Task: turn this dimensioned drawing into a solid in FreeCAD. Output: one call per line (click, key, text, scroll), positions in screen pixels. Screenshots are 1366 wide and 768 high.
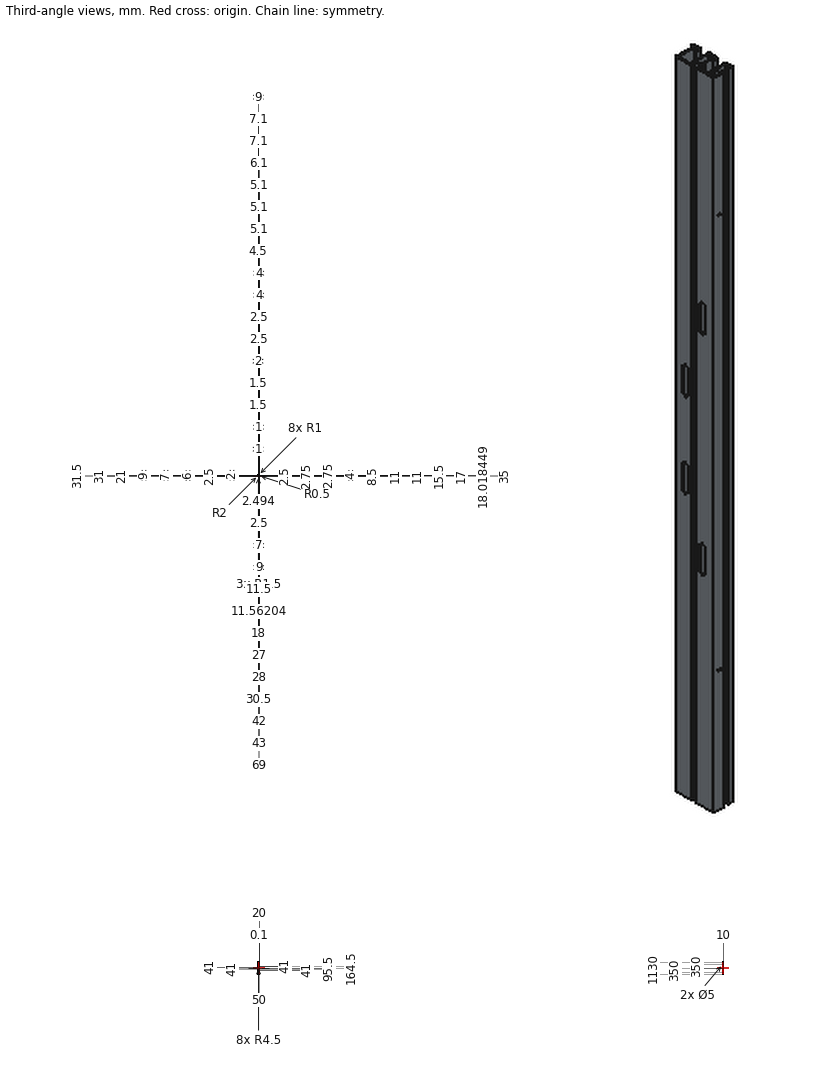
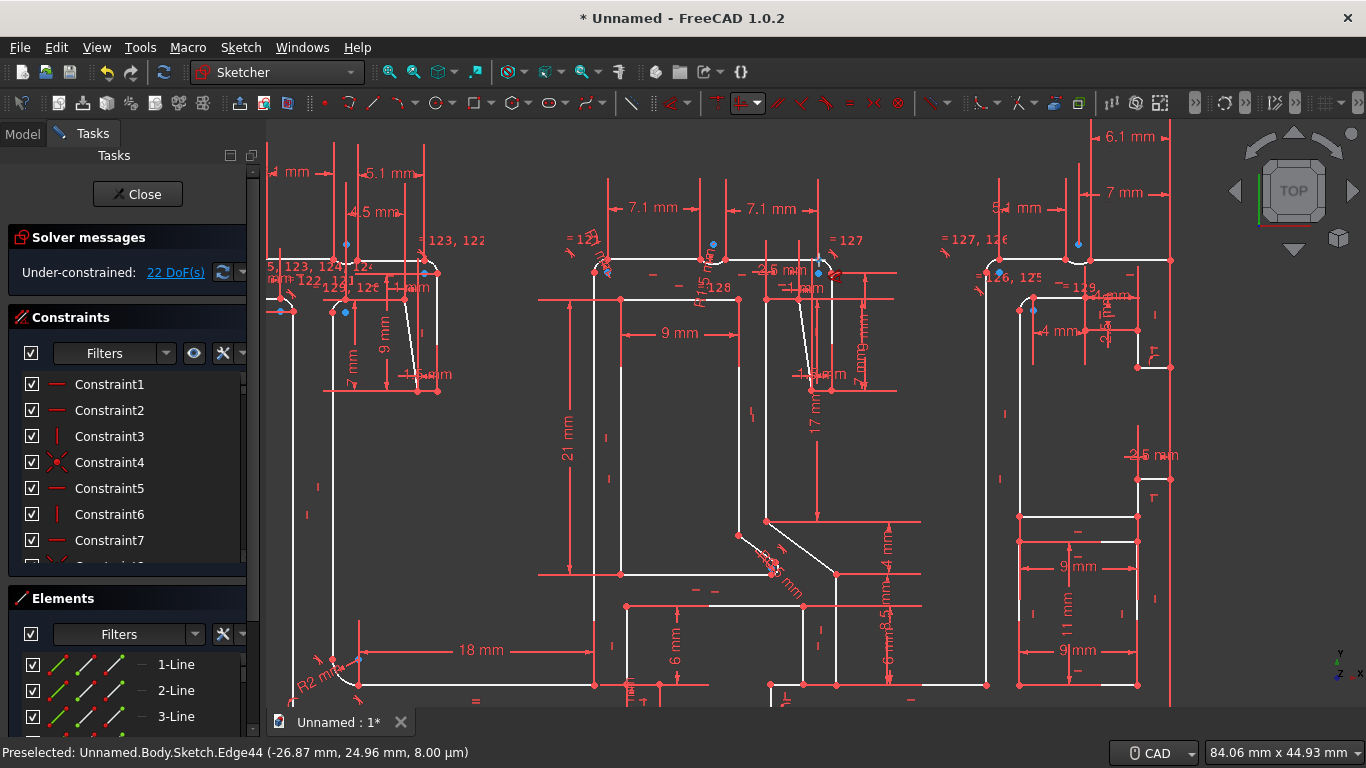
click(818, 260)
click(914, 226)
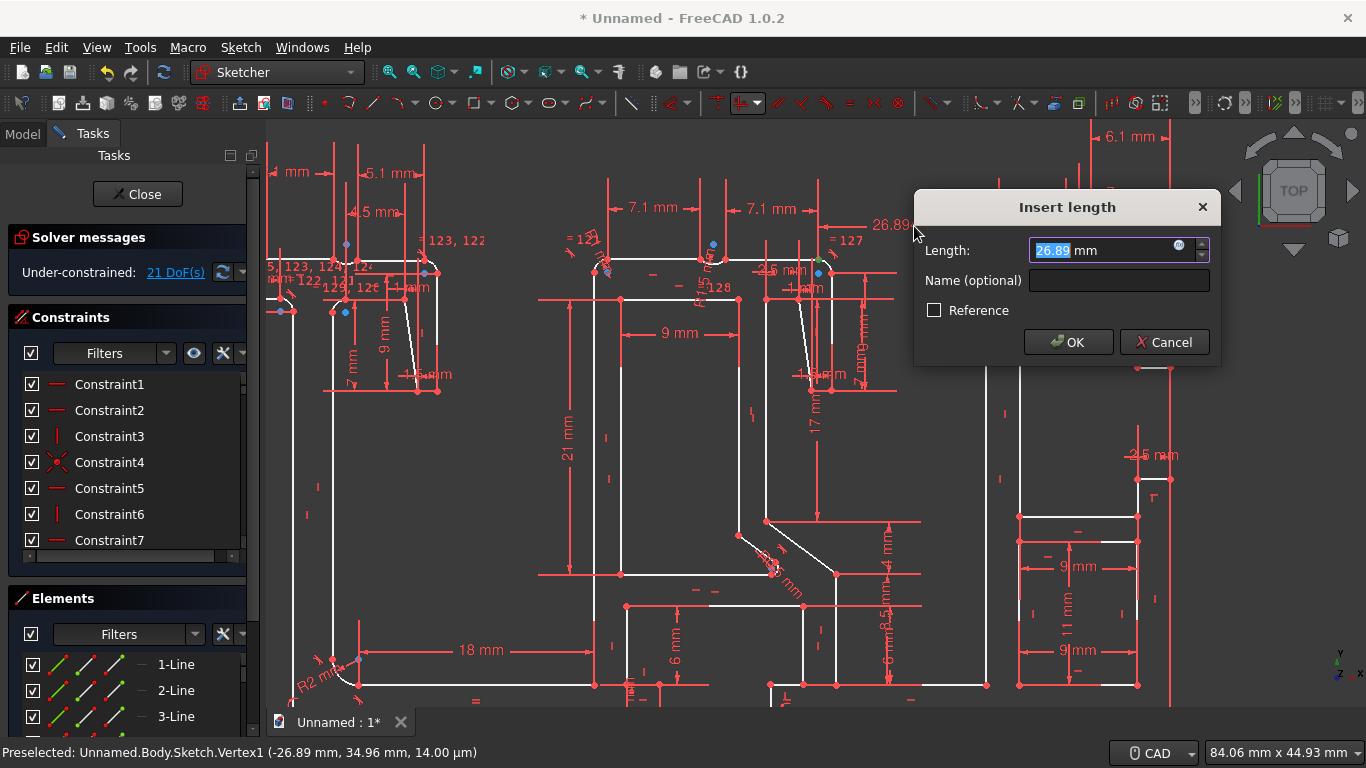
text(27)
key(Return)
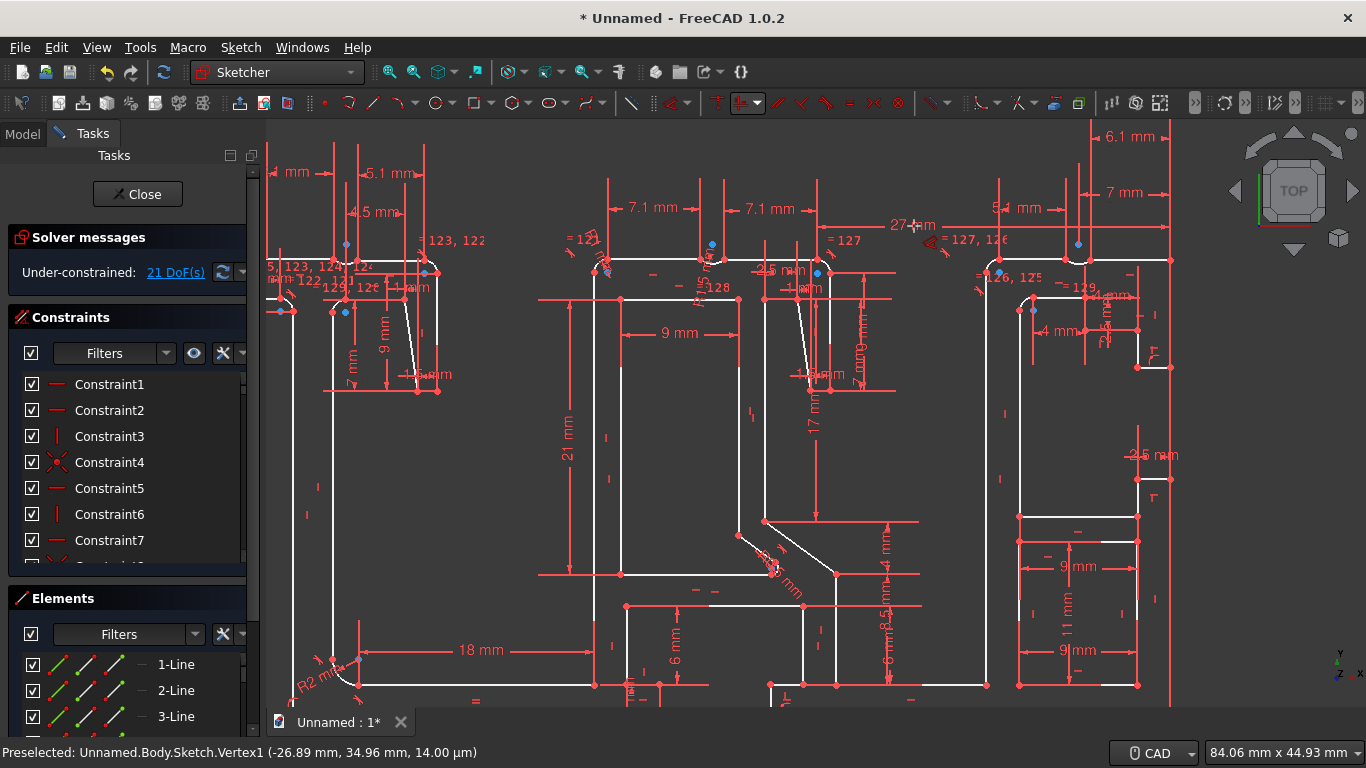
click(817, 260)
click(783, 469)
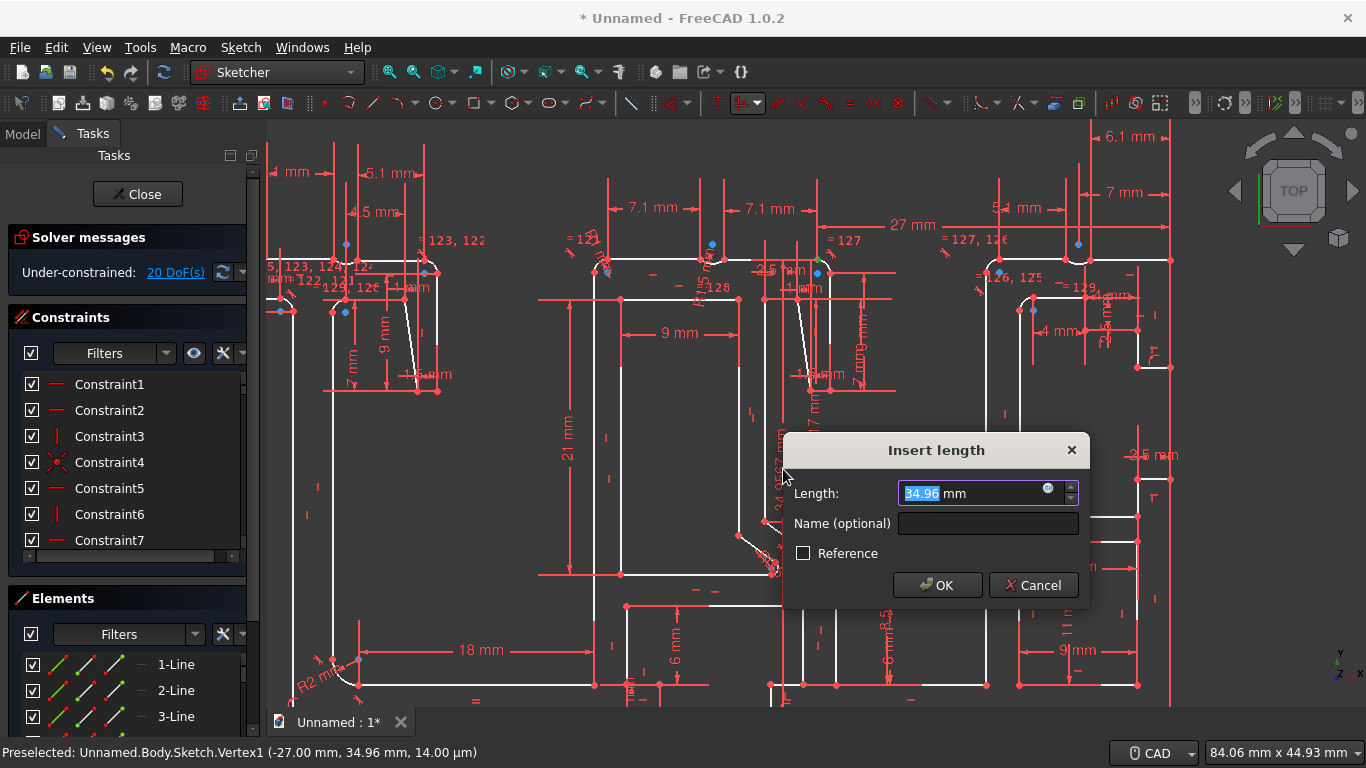
text(35)
key(Return)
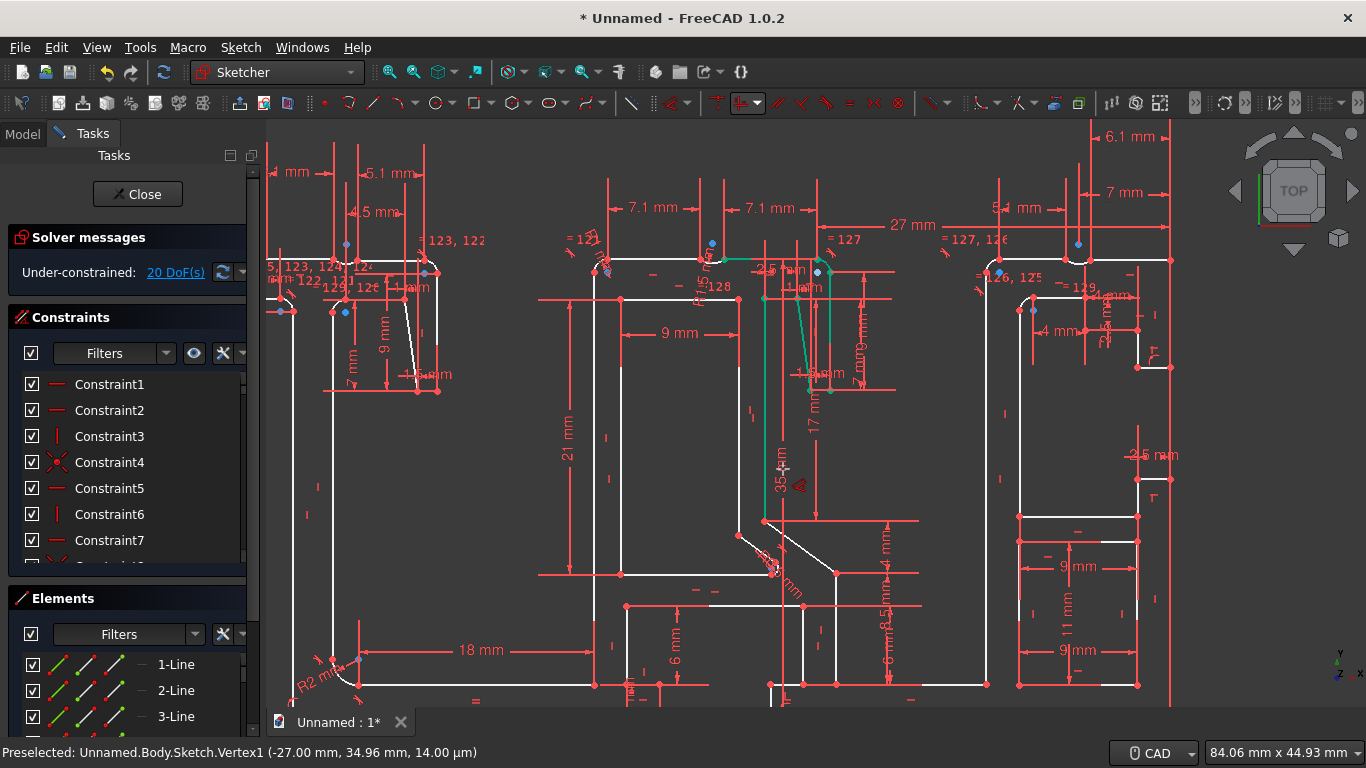
click(700, 259)
click(666, 469)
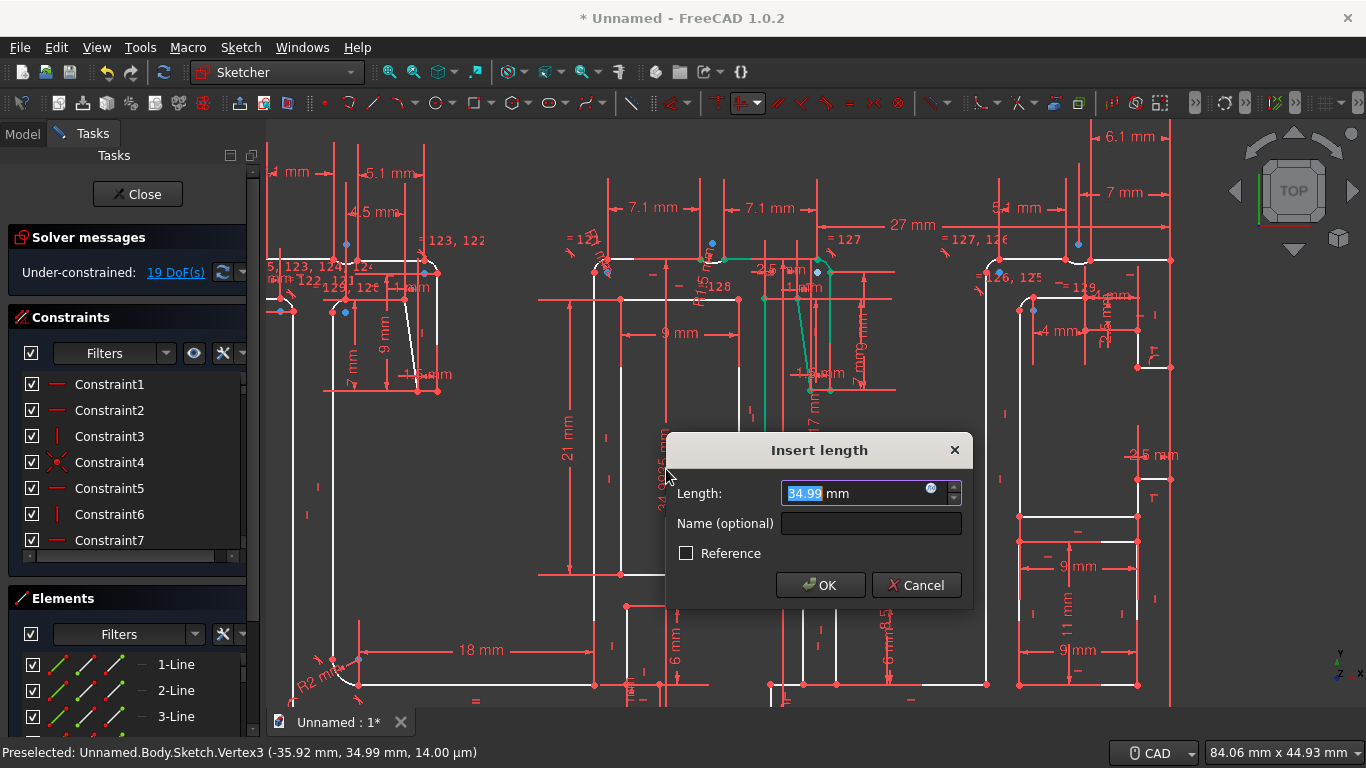
text(35)
key(Return)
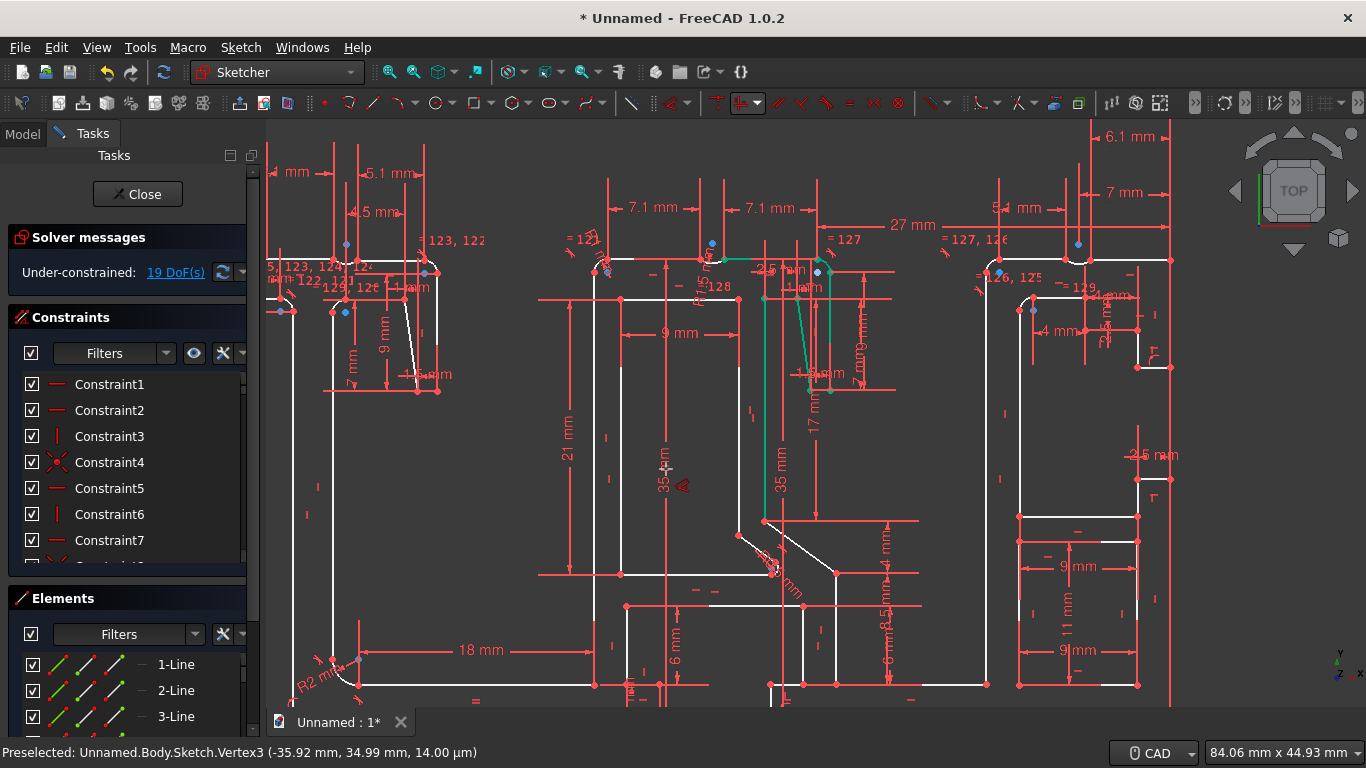
click(608, 259)
click(889, 201)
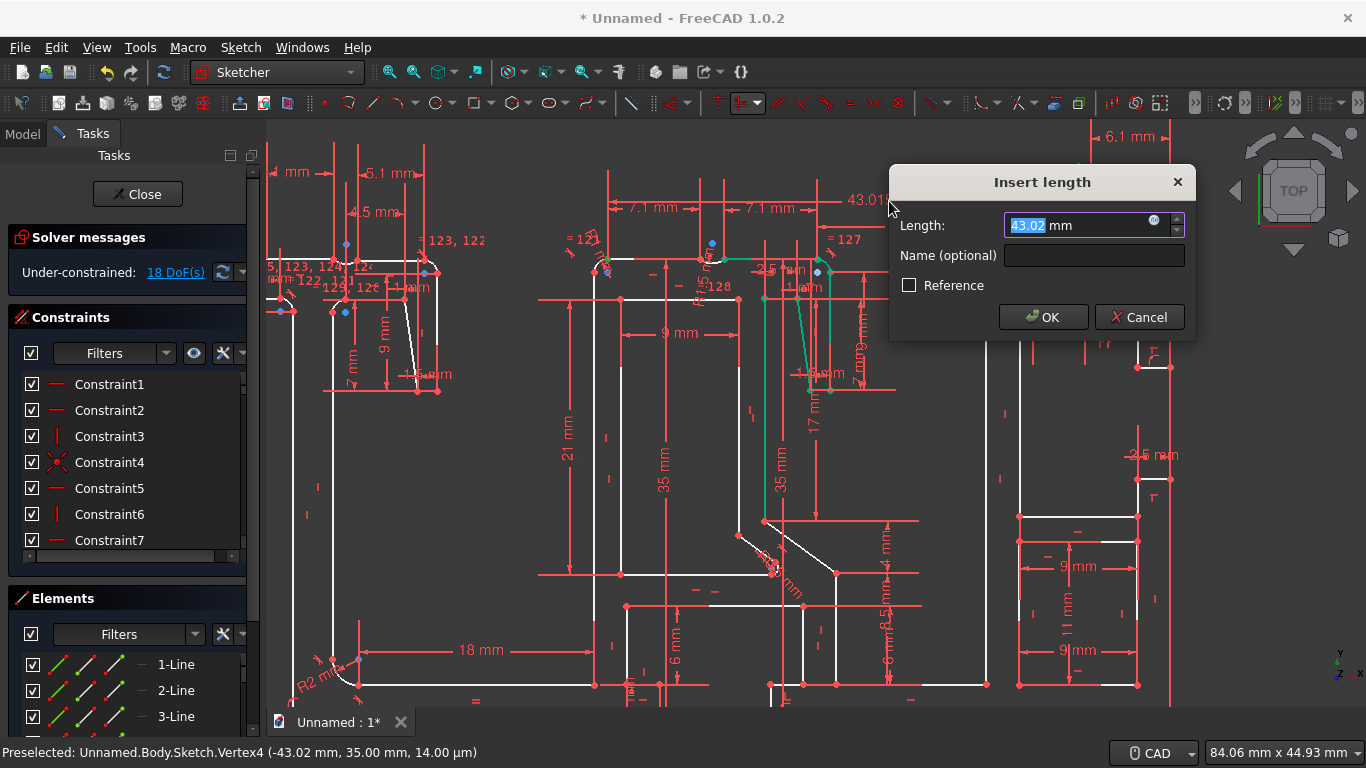
text(43)
key(Return)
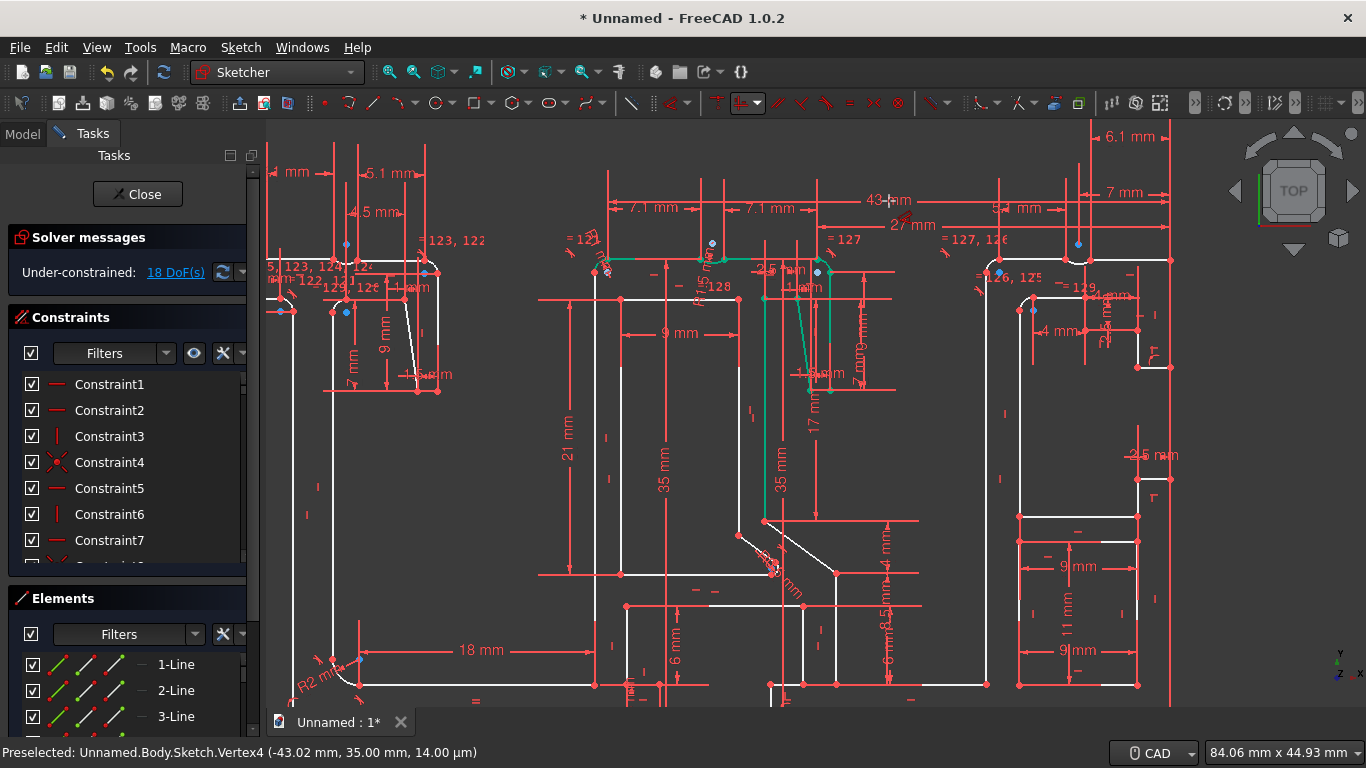
click(333, 313)
click(299, 496)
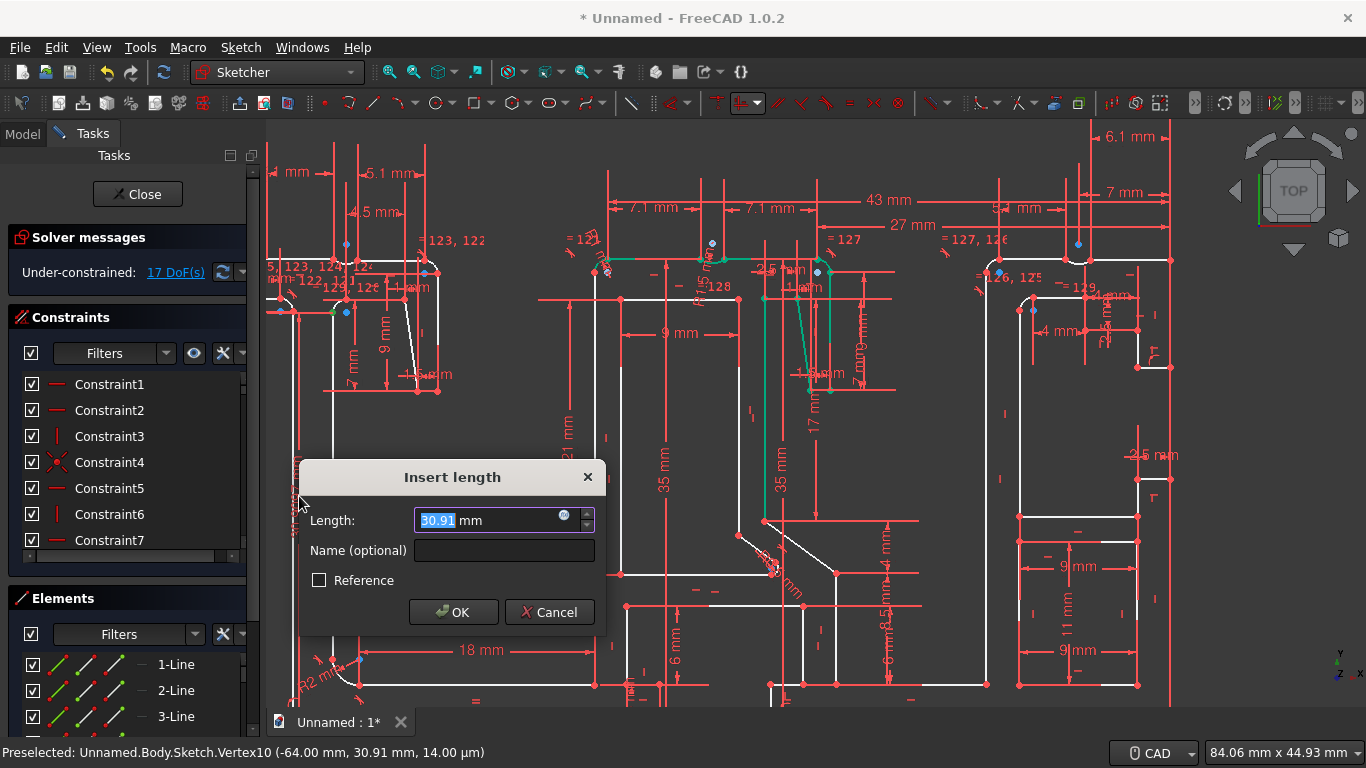
text(31)
key(Return)